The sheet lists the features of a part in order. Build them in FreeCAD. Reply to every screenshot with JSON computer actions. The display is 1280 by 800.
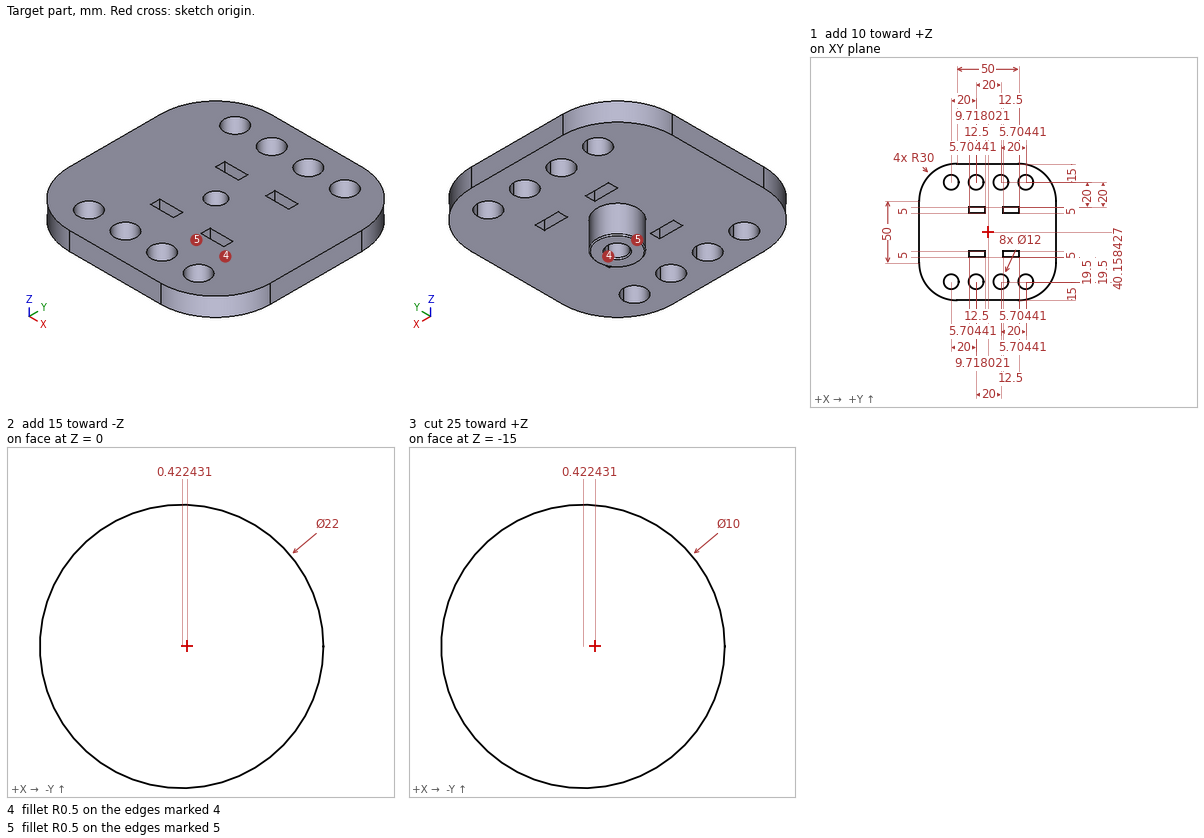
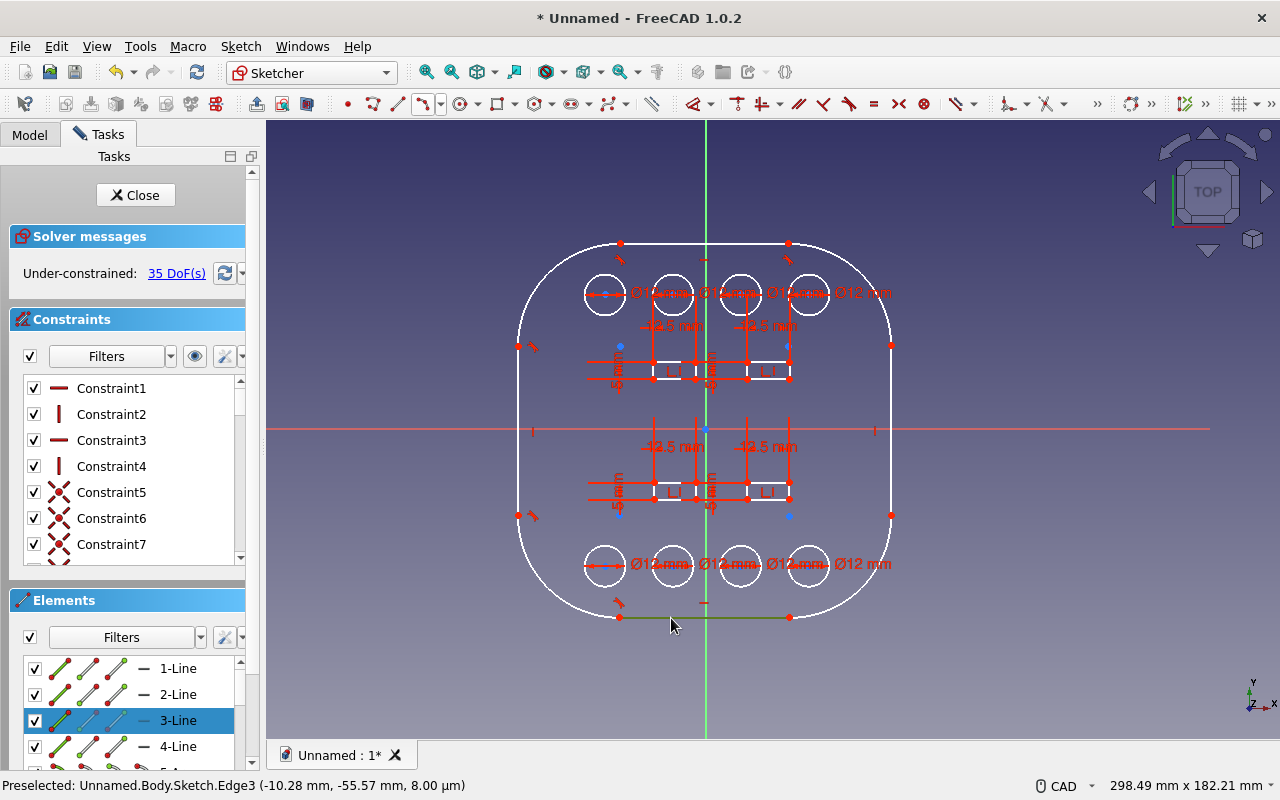
{"action": "left_click", "coordinate": [835, 607]}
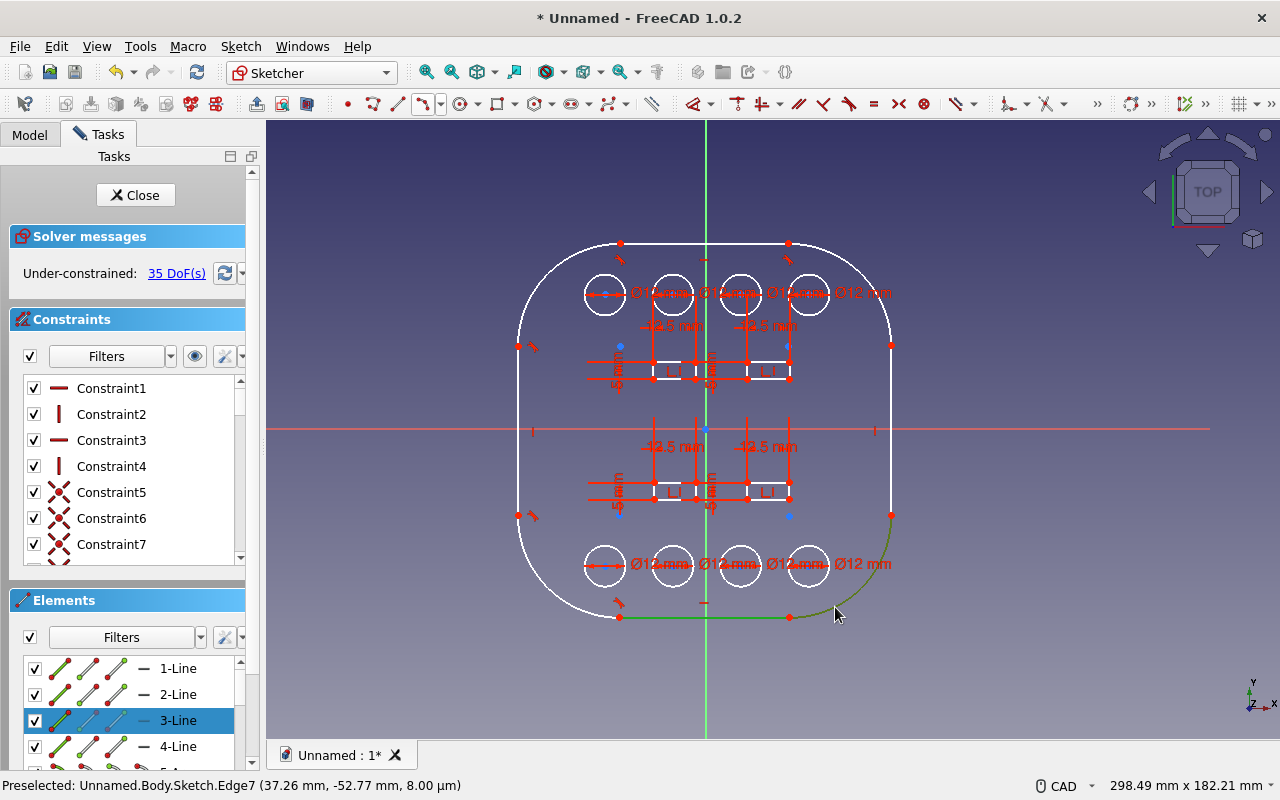
{"action": "key", "text": "t"}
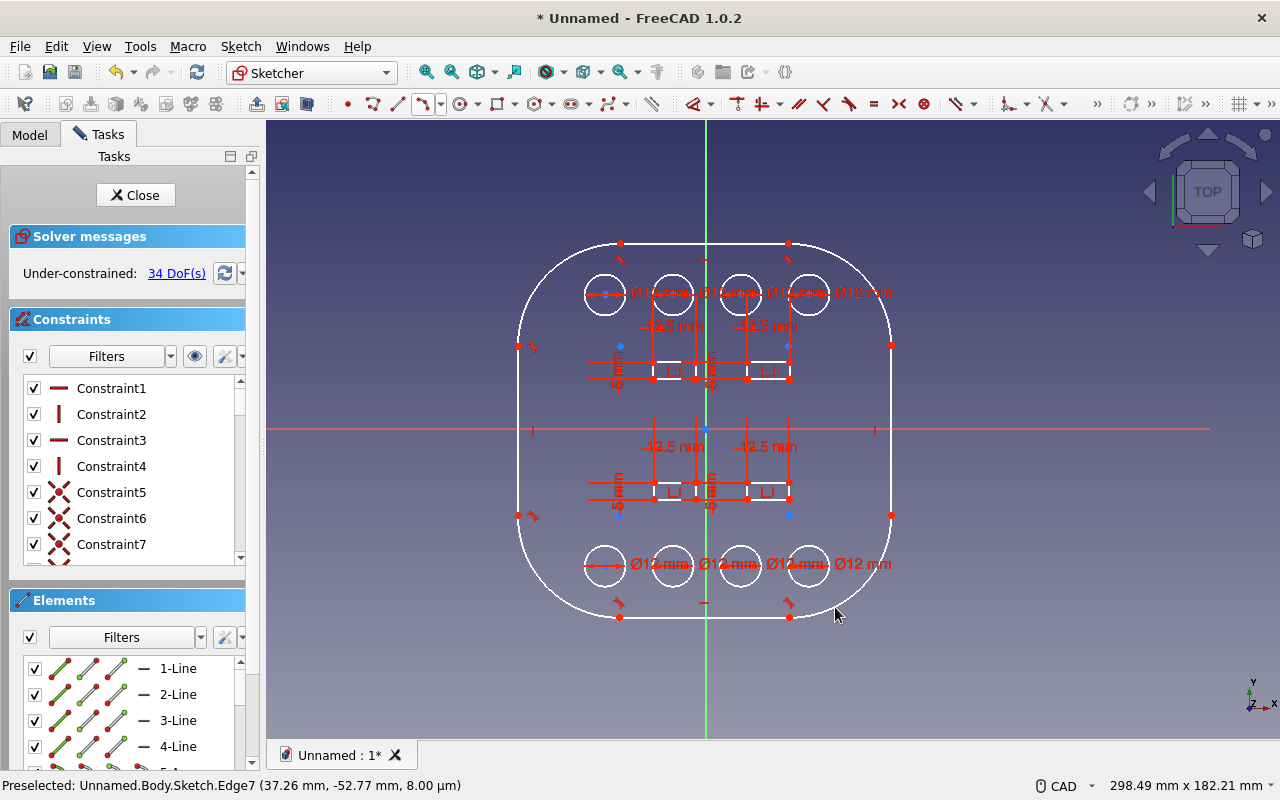
{"action": "left_click", "coordinate": [891, 465]}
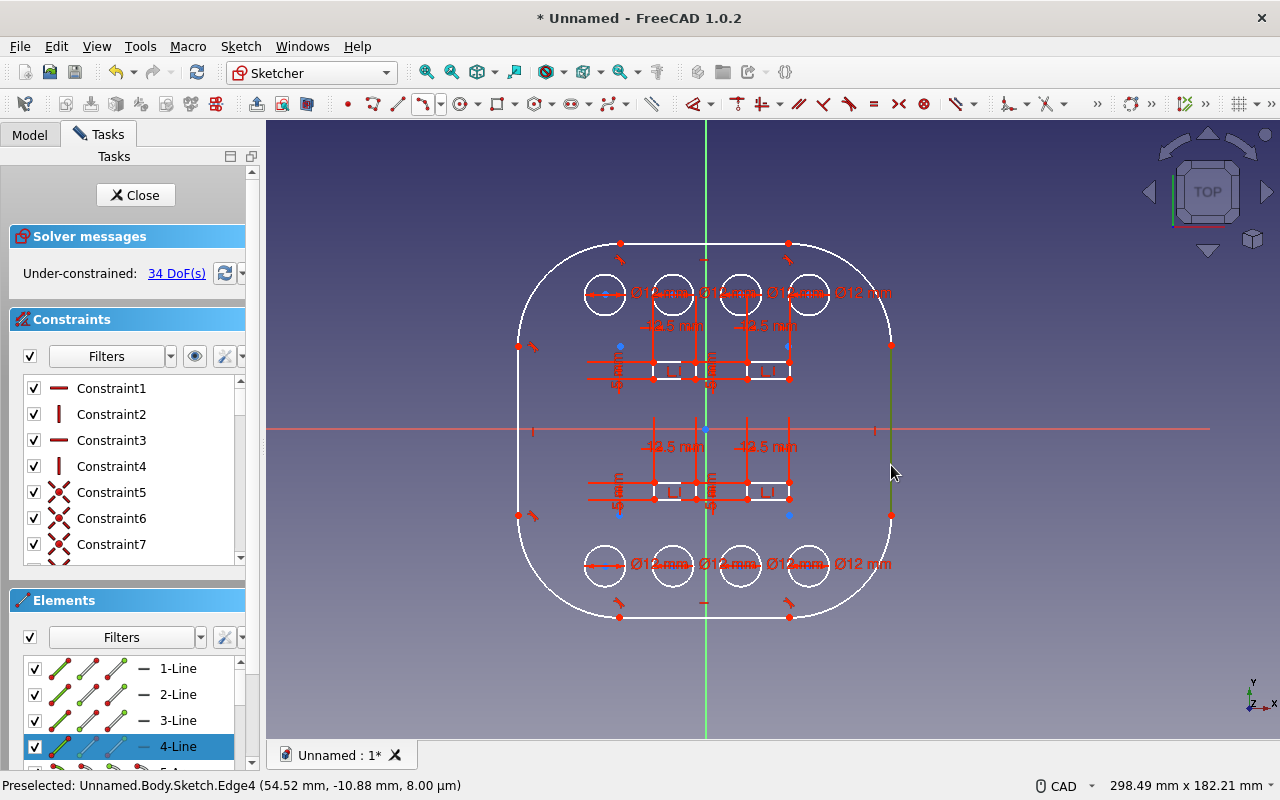
{"action": "left_click", "coordinate": [835, 607]}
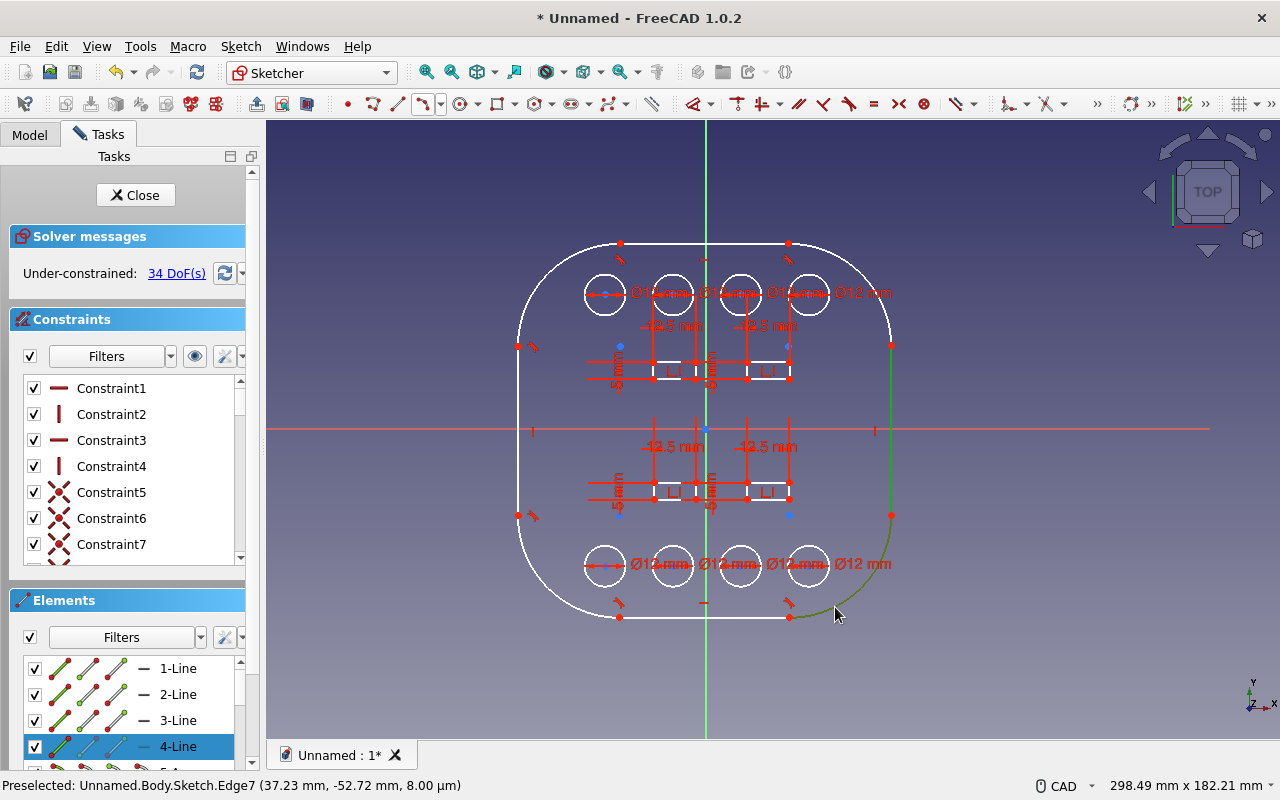
{"action": "left_click", "coordinate": [849, 104]}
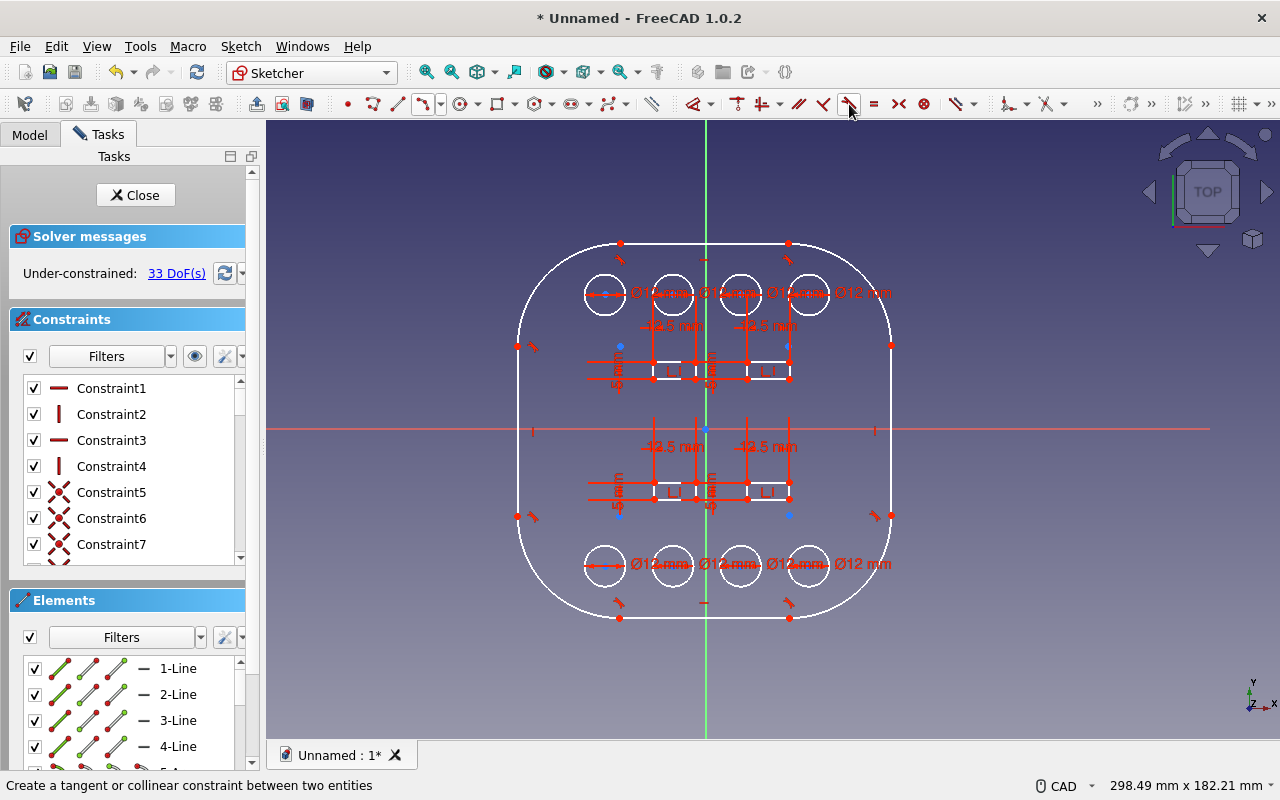
{"action": "left_click", "coordinate": [891, 465]}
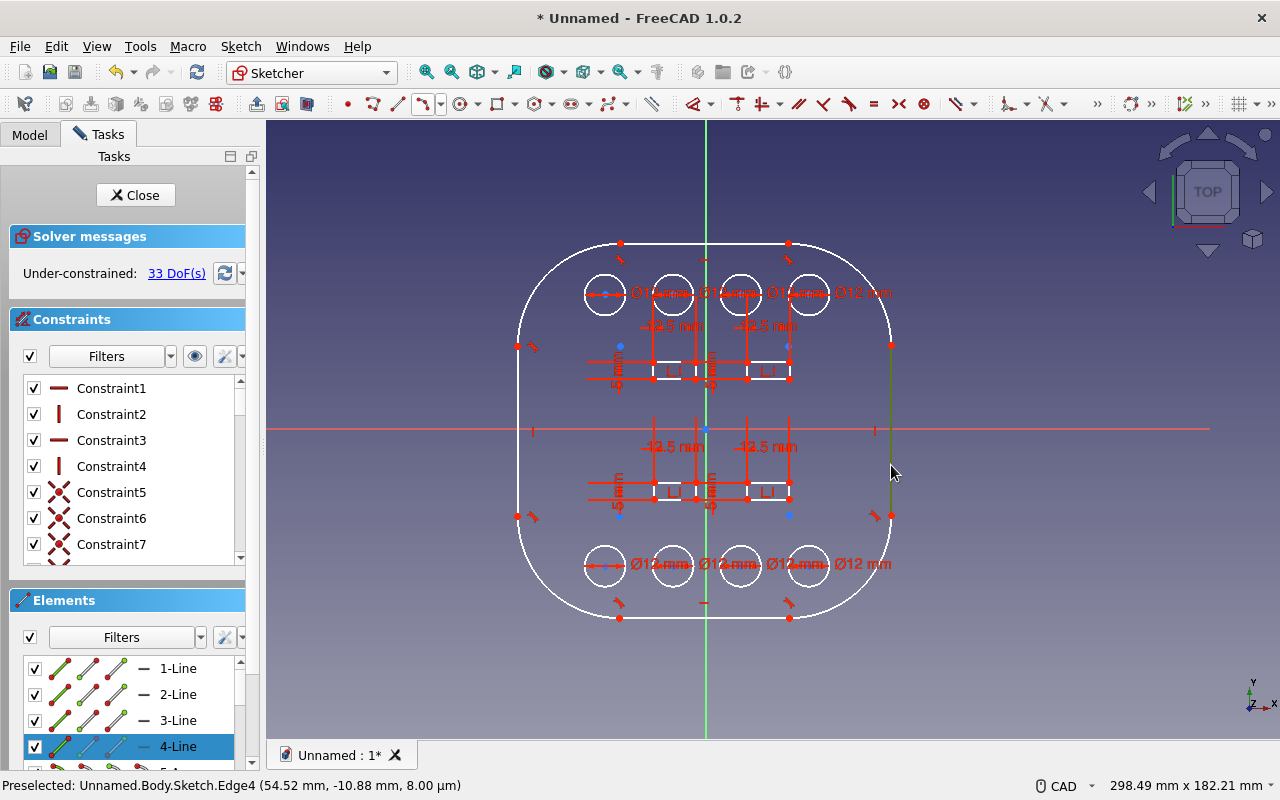
{"action": "left_click", "coordinate": [880, 300]}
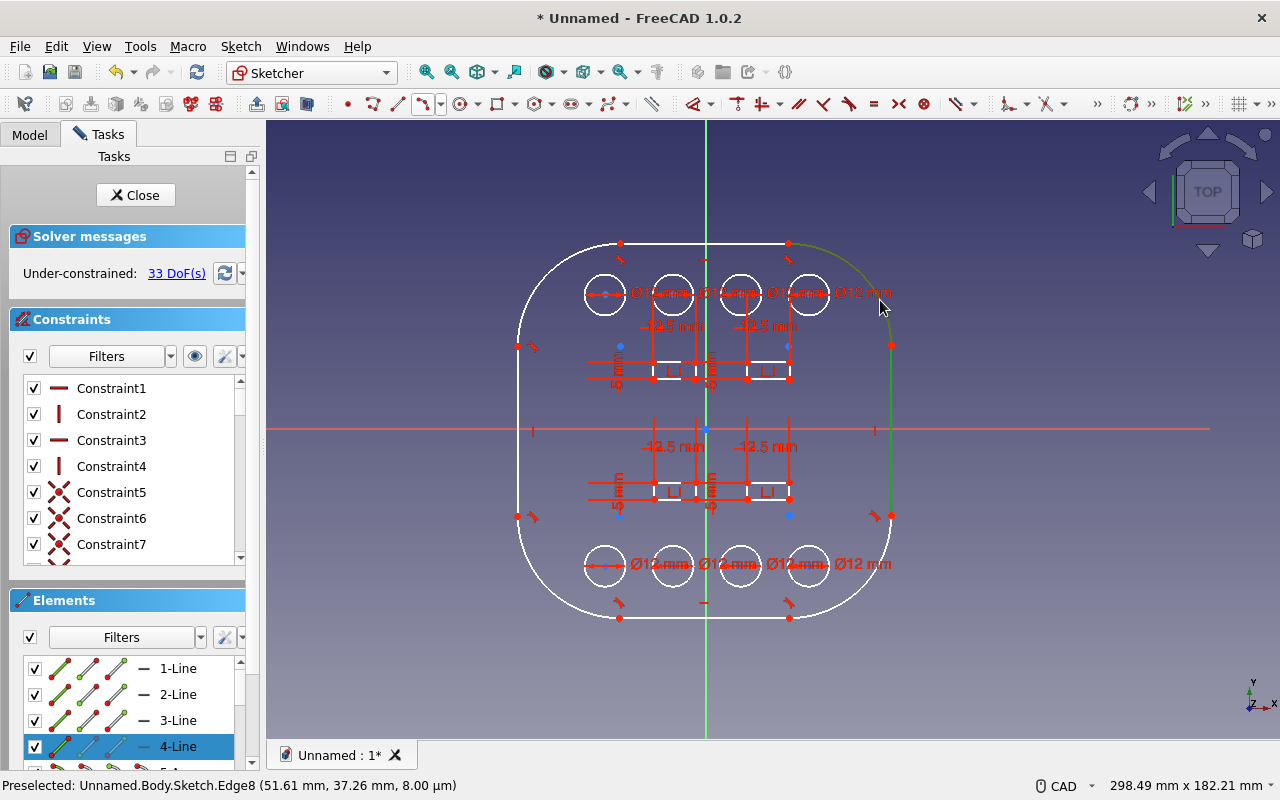
{"action": "left_click", "coordinate": [849, 104]}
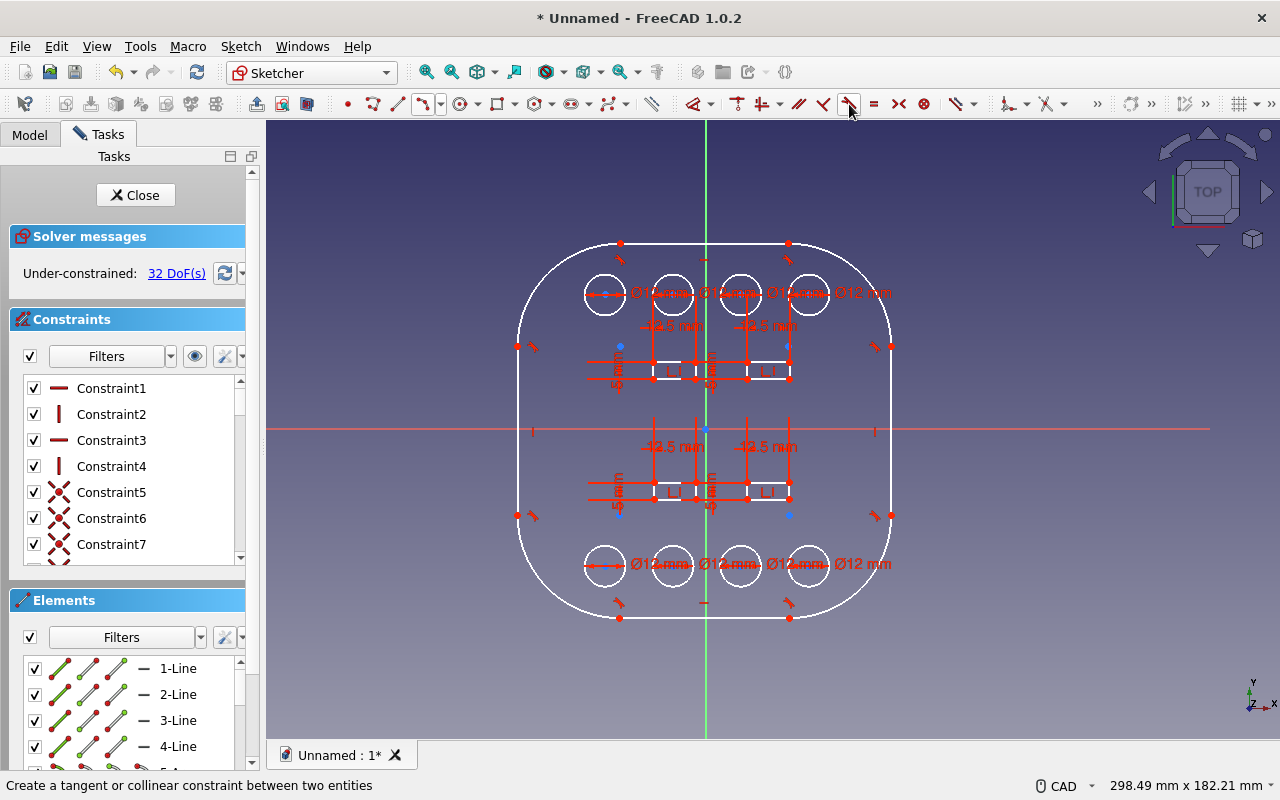
{"action": "left_click", "coordinate": [574, 255]}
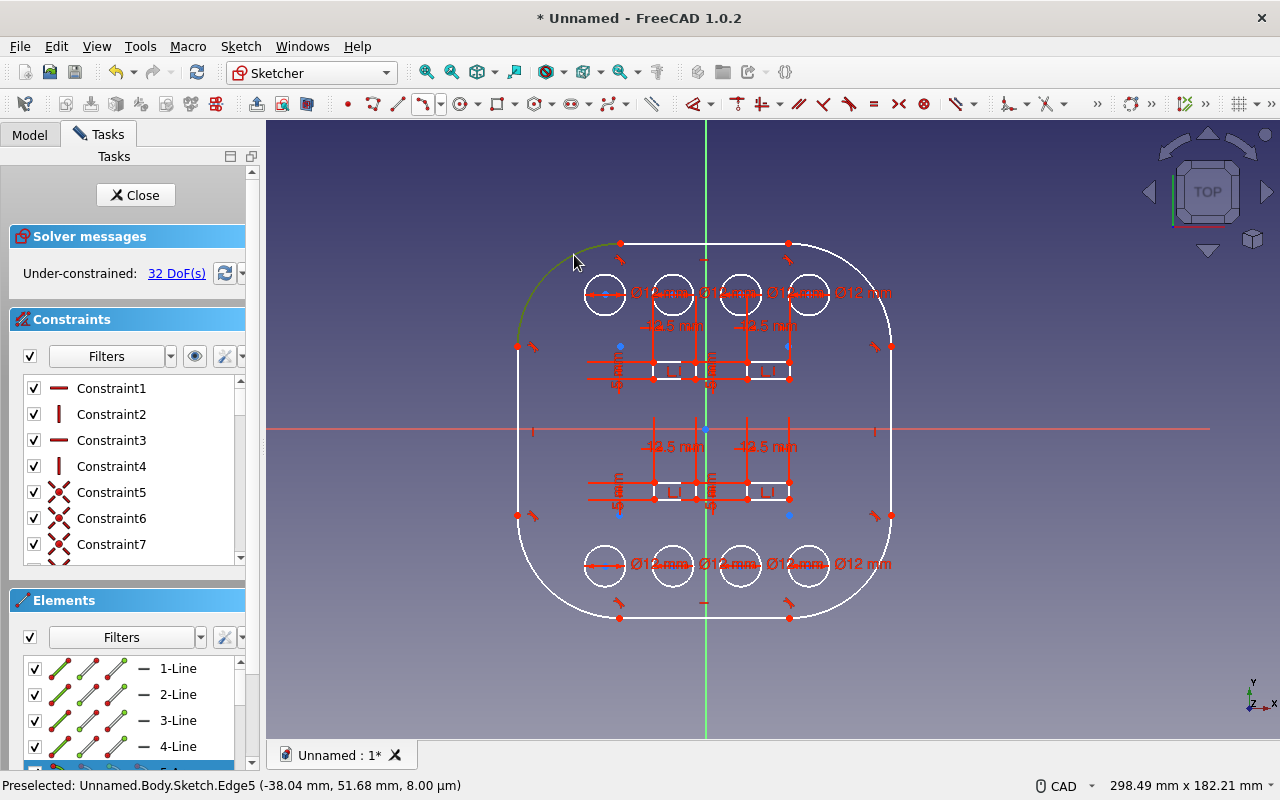
{"action": "left_click", "coordinate": [529, 562]}